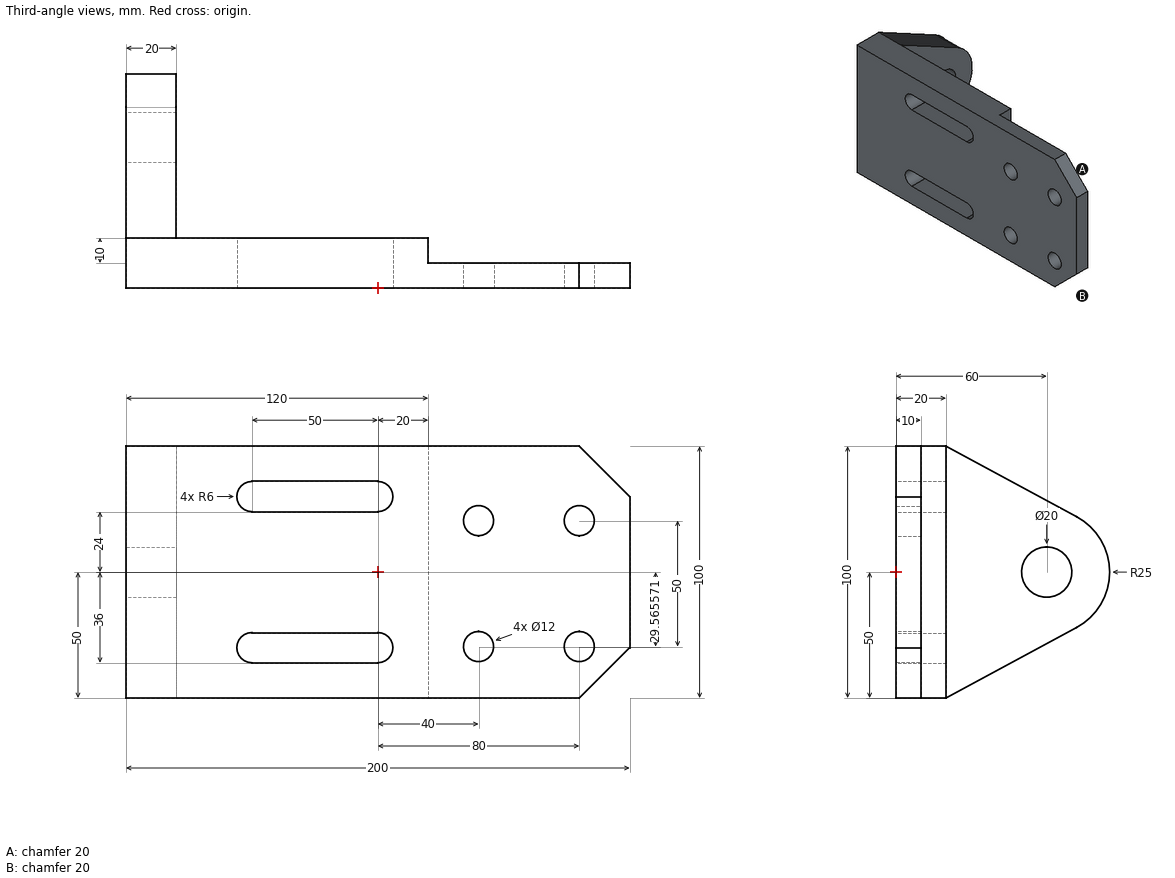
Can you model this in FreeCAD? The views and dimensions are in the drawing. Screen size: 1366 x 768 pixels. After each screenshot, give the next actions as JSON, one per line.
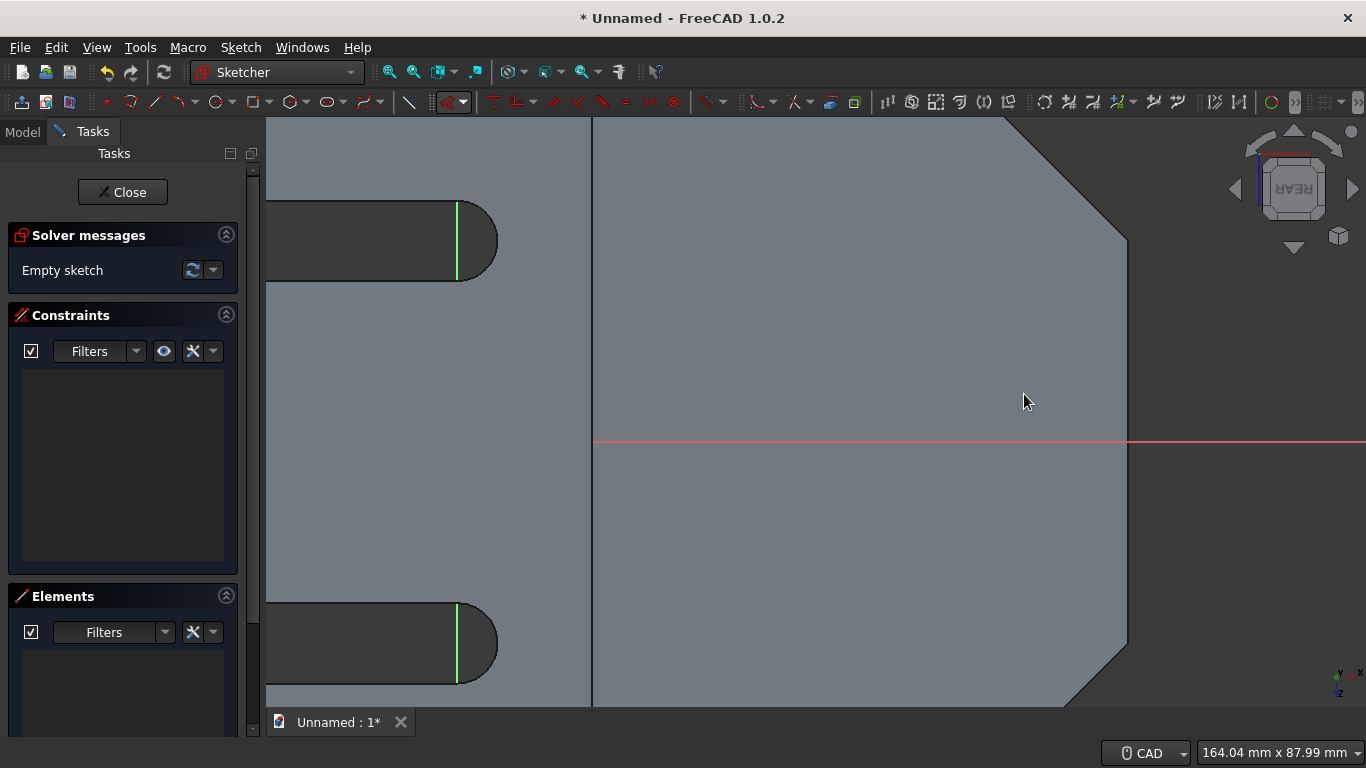
{"action": "left_click", "coordinate": [216, 102]}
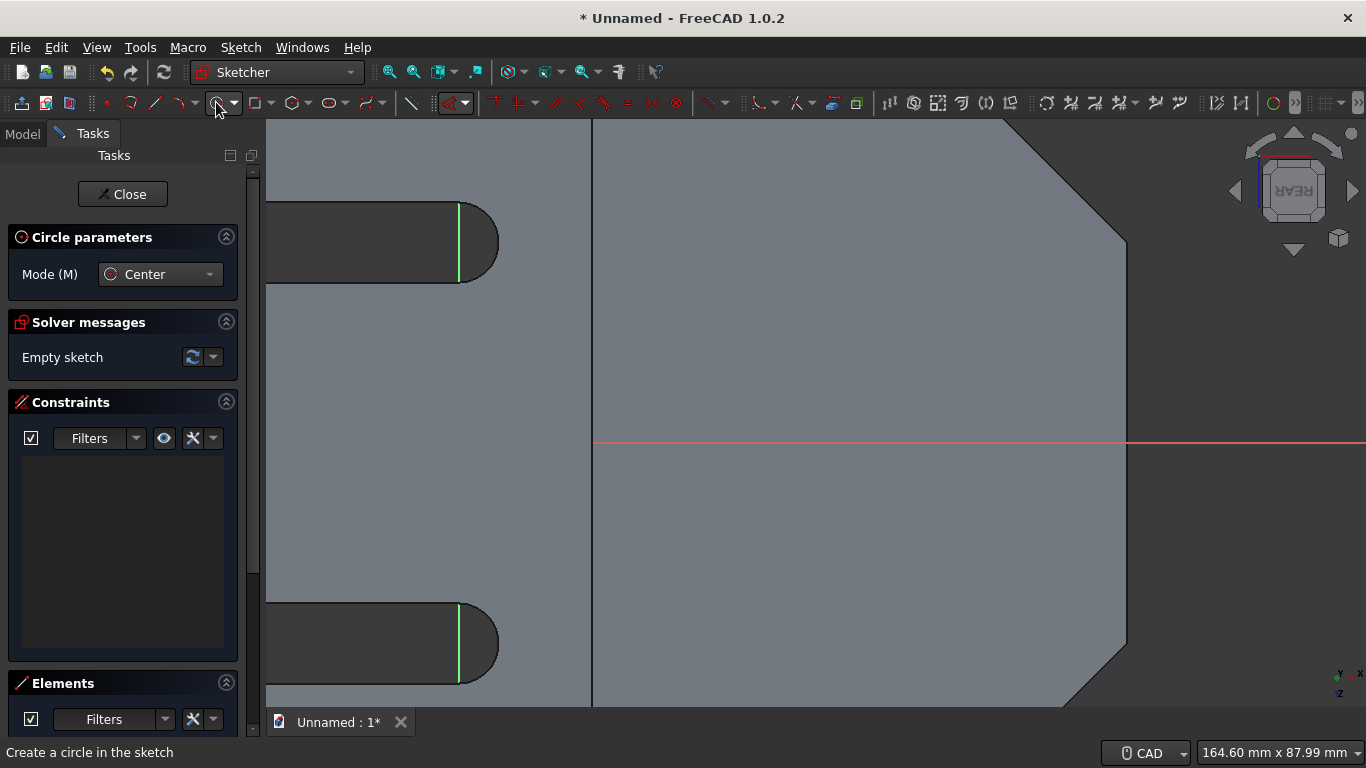
{"action": "left_click", "coordinate": [726, 245]}
{"action": "mouse_move", "coordinate": [754, 217]}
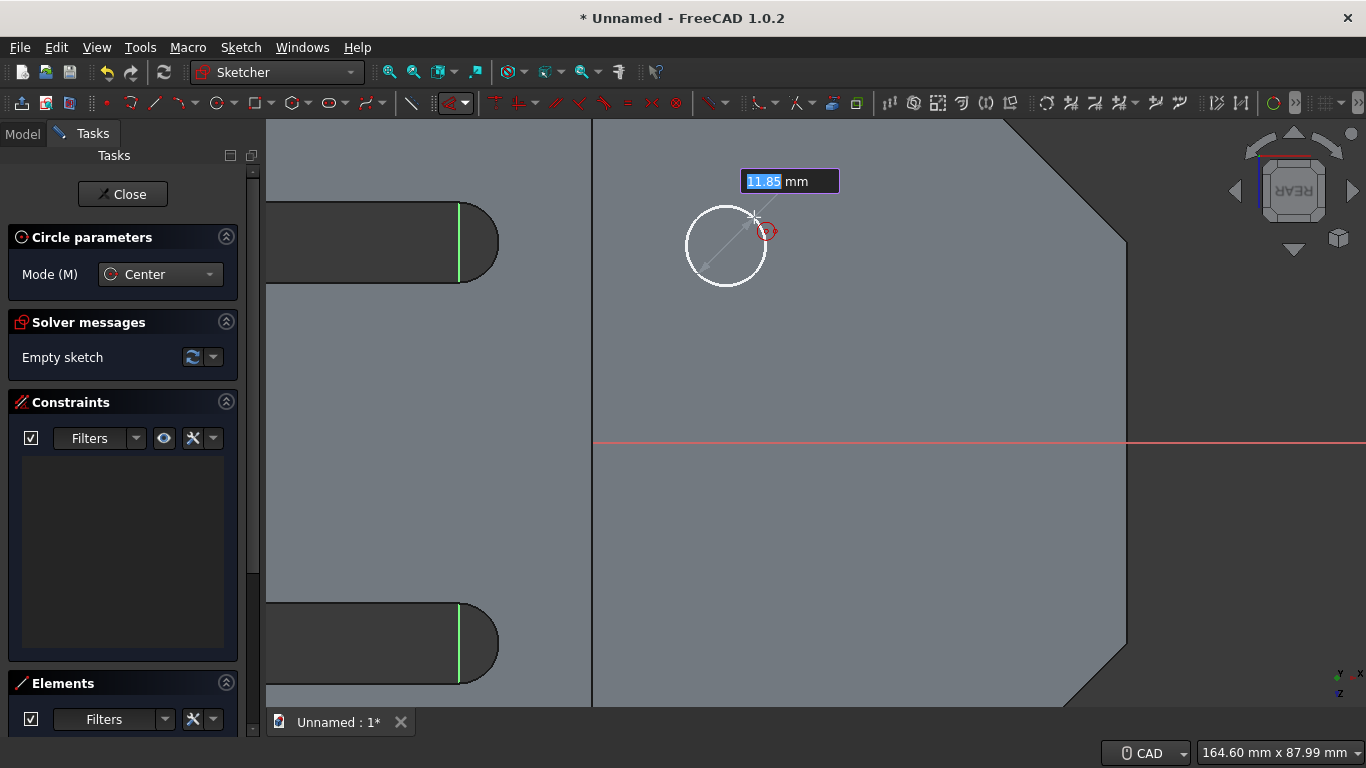
{"action": "type", "text": "12"}
{"action": "key", "text": "Return"}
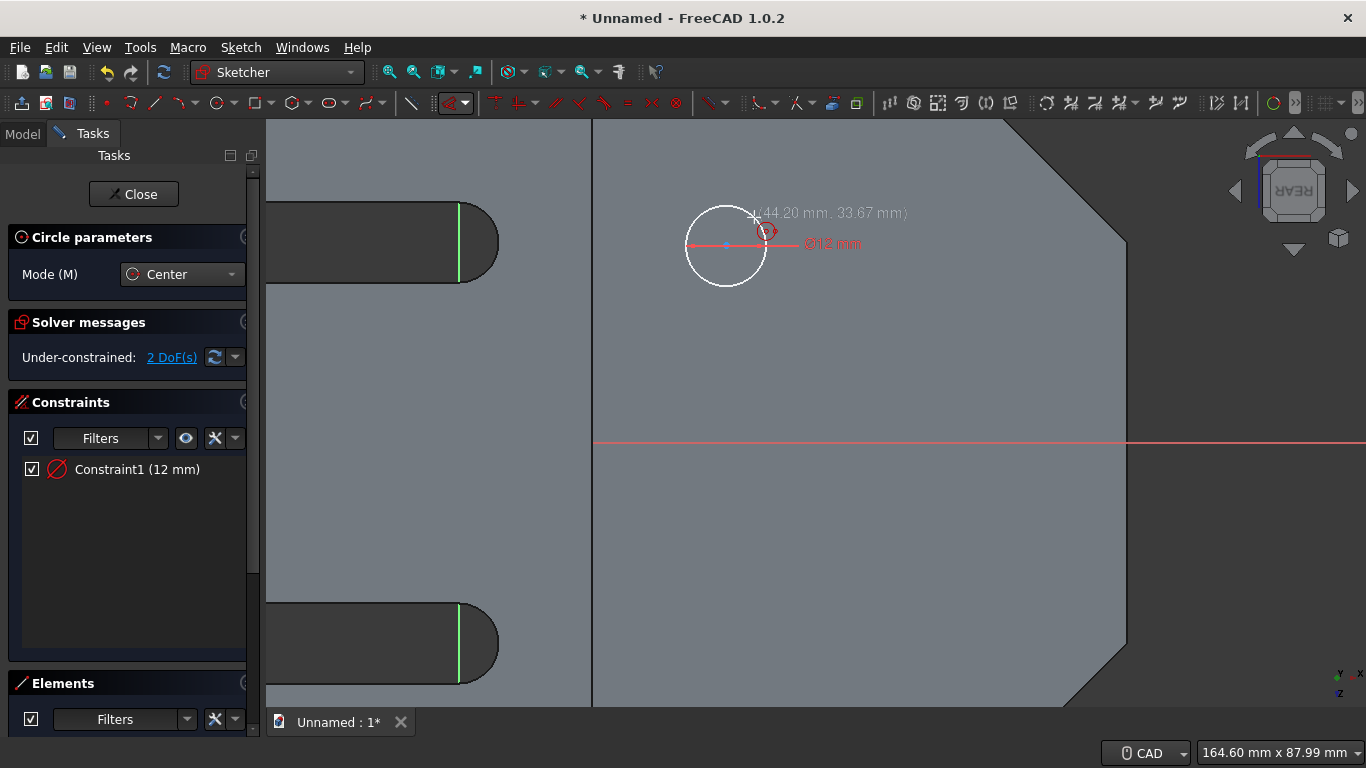
{"action": "left_click", "coordinate": [993, 245]}
{"action": "mouse_move", "coordinate": [1022, 217]}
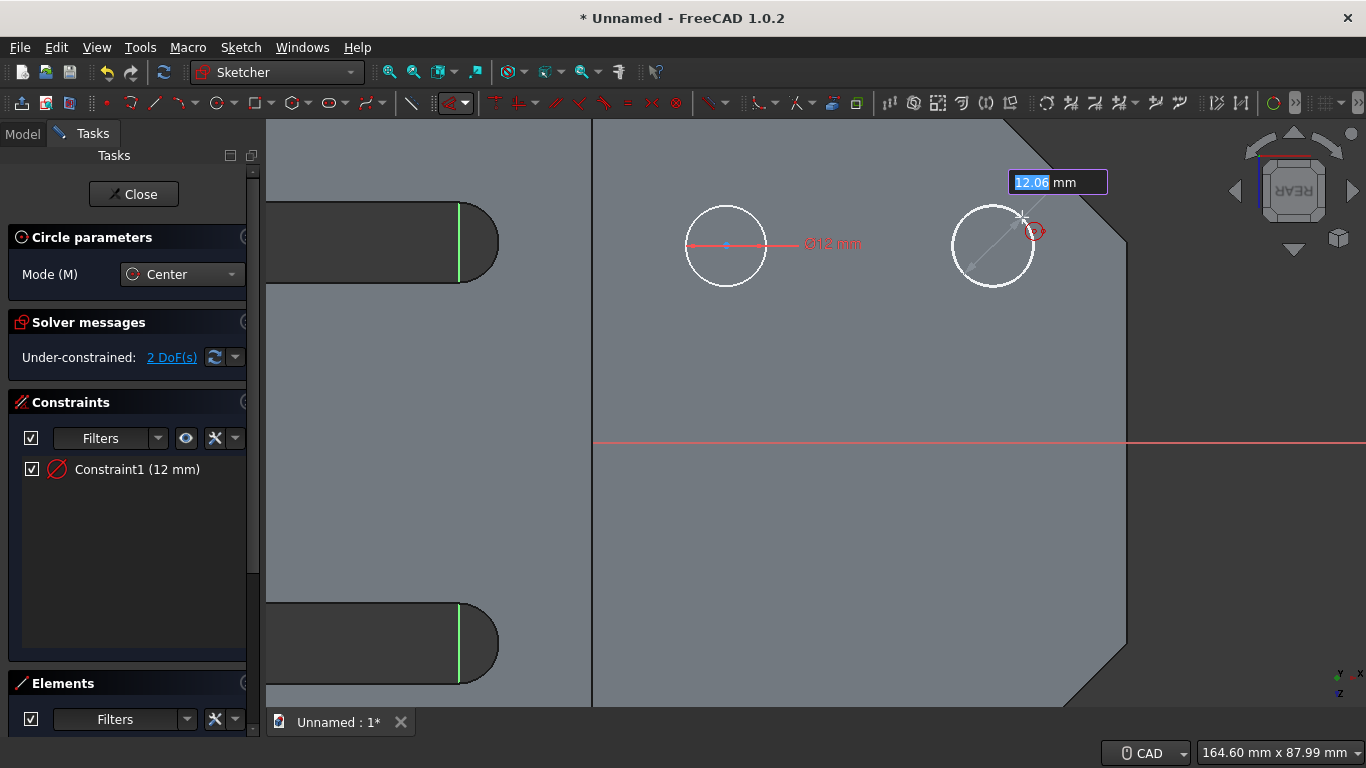
{"action": "type", "text": "12"}
{"action": "key", "text": "Return"}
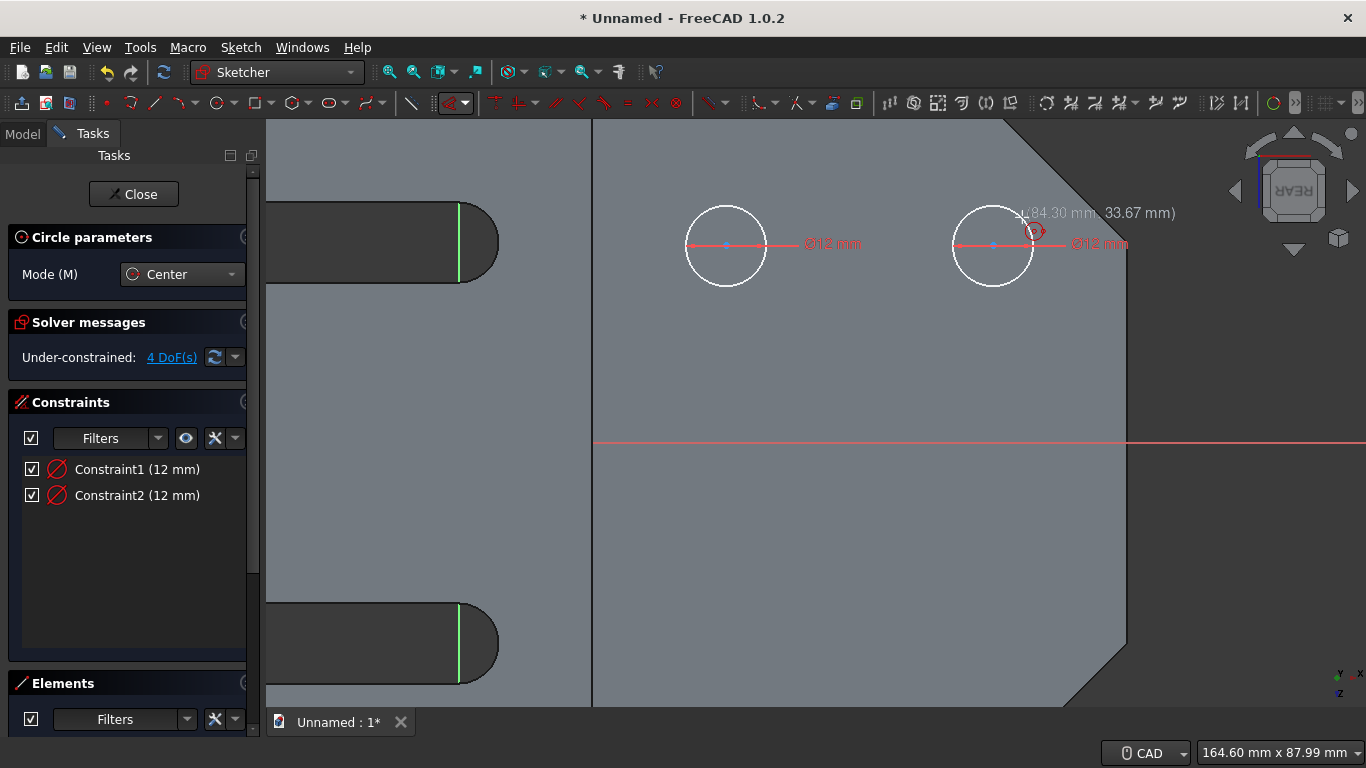
{"action": "left_click", "coordinate": [993, 580]}
{"action": "mouse_move", "coordinate": [1022, 551]}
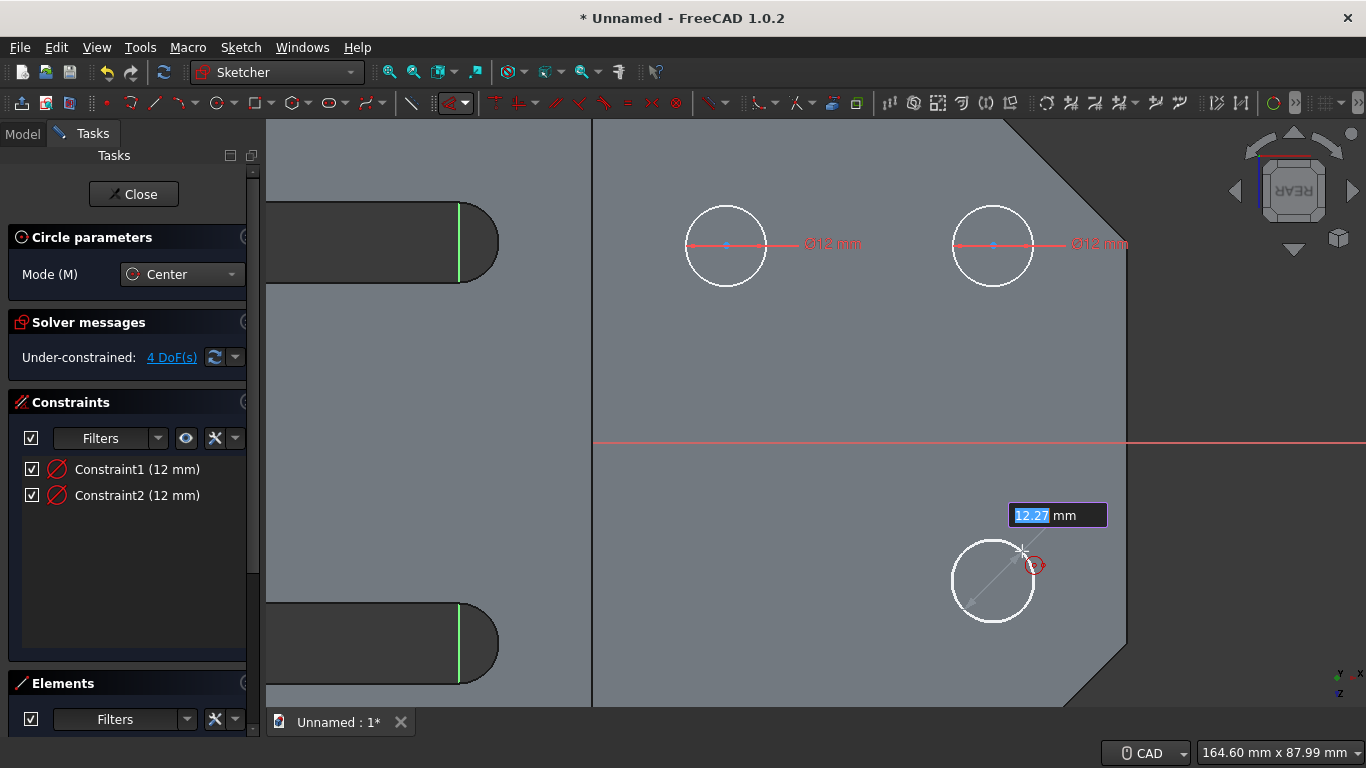
{"action": "type", "text": "12"}
{"action": "key", "text": "Return"}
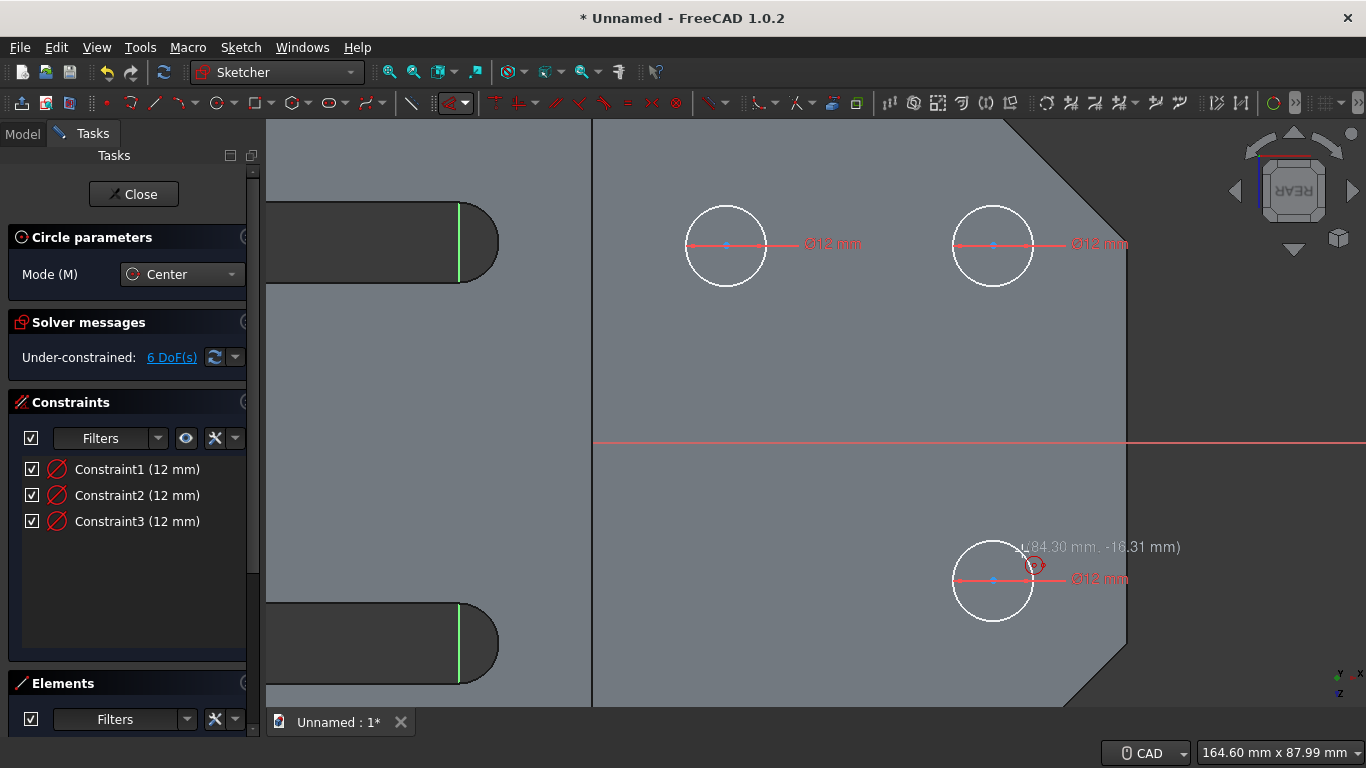
{"action": "left_click", "coordinate": [726, 580]}
{"action": "mouse_move", "coordinate": [754, 551]}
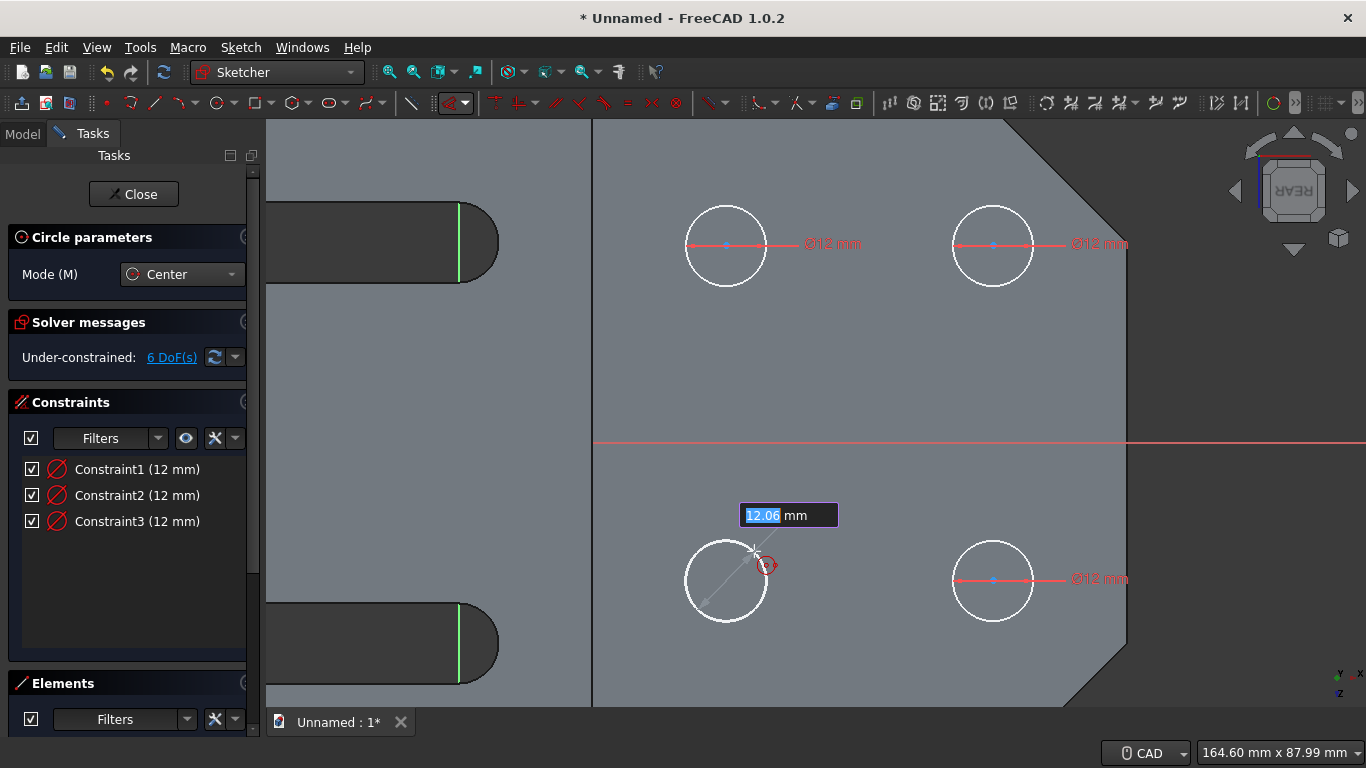
{"action": "type", "text": "12"}
{"action": "key", "text": "Return"}
{"action": "key", "text": "Escape"}